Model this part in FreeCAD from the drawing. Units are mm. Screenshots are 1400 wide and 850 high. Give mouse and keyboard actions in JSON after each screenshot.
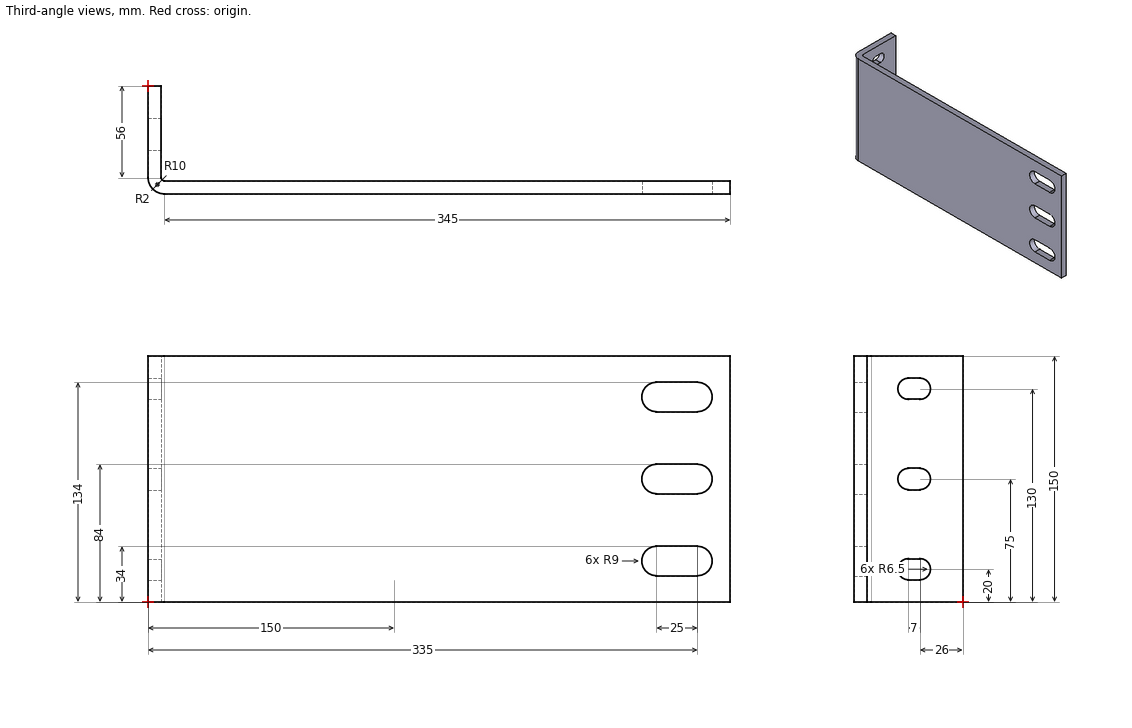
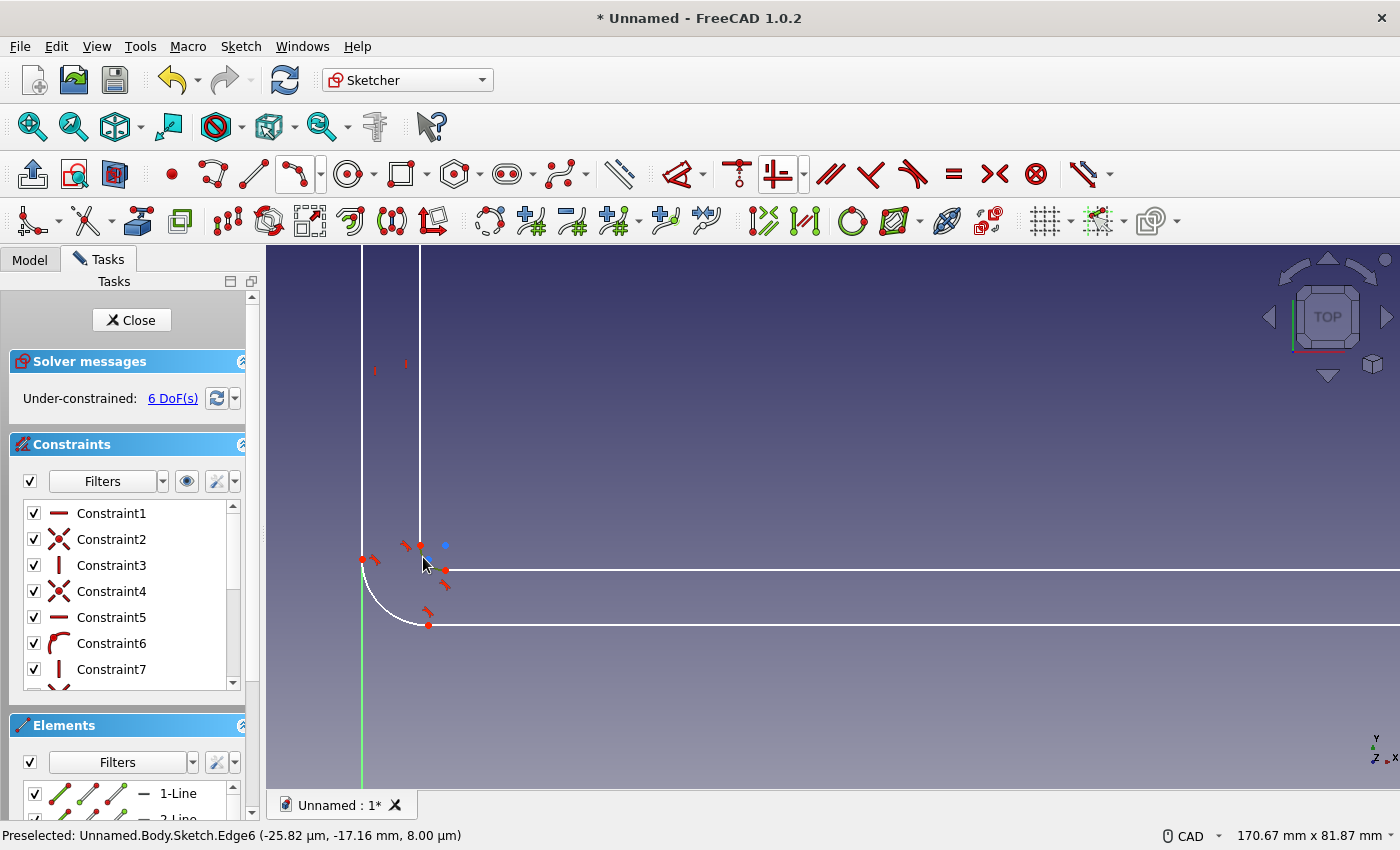
{"action": "left_click", "coordinate": [398, 618]}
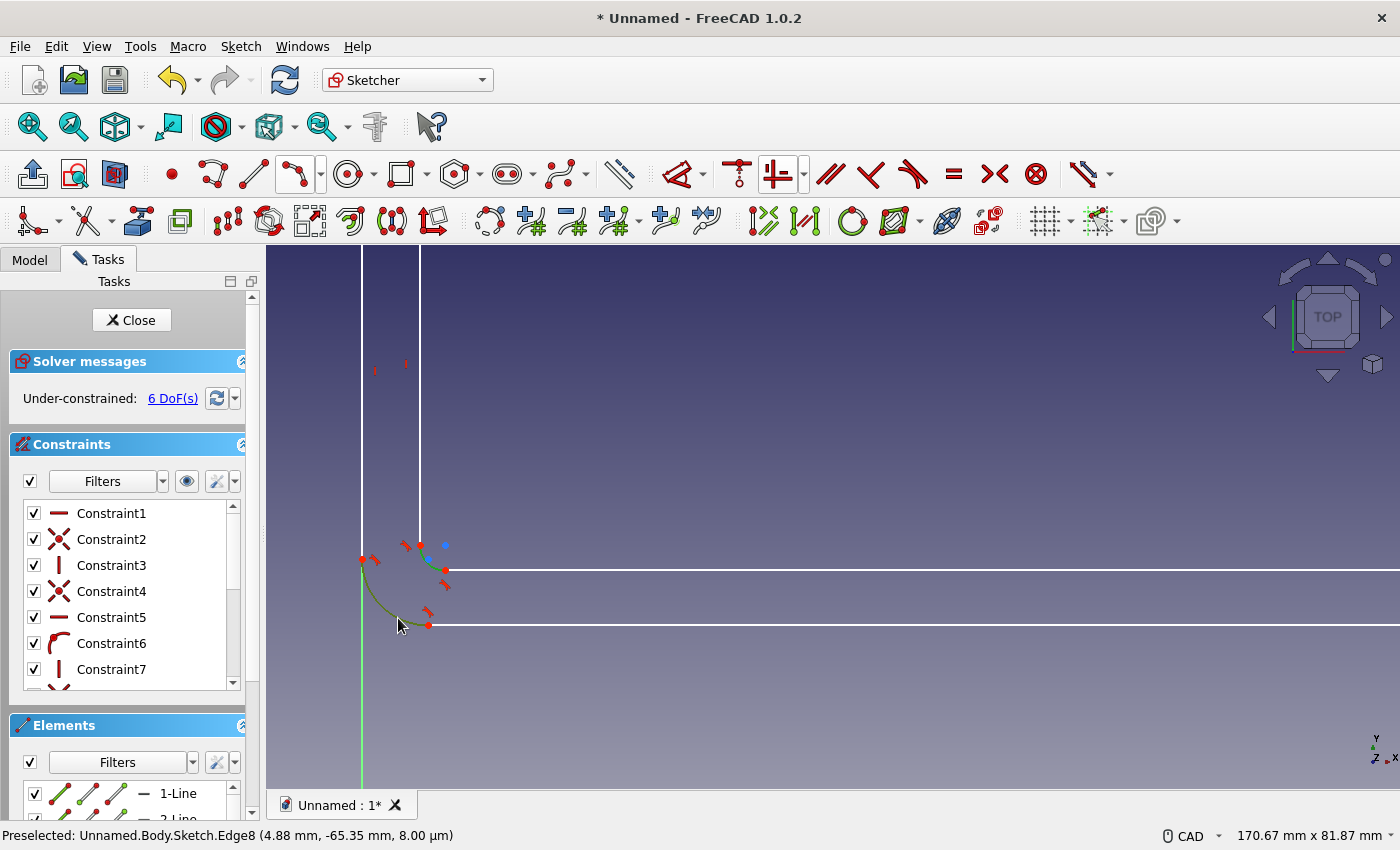
{"action": "left_click", "coordinate": [737, 174]}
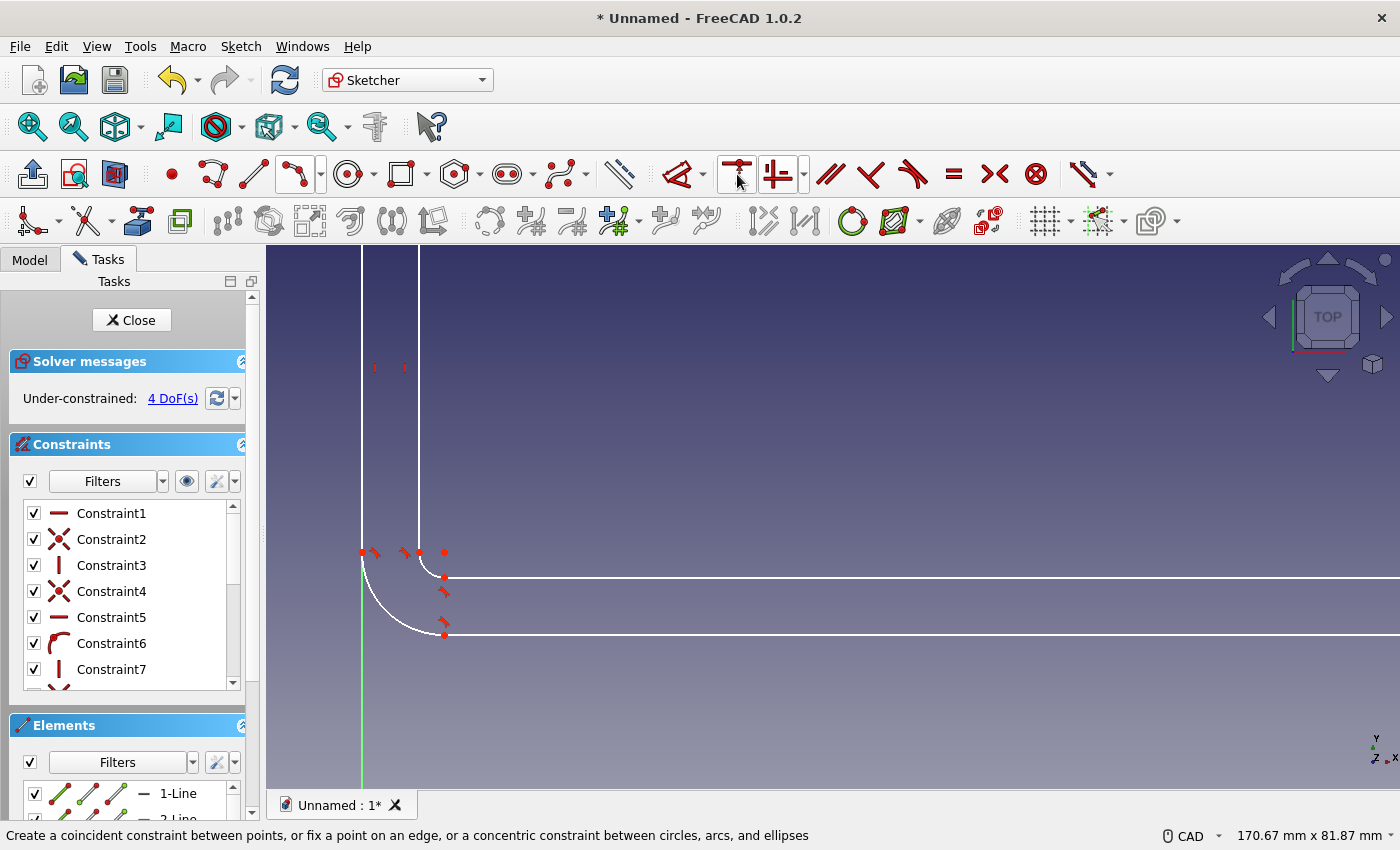
{"action": "left_click", "coordinate": [676, 174]}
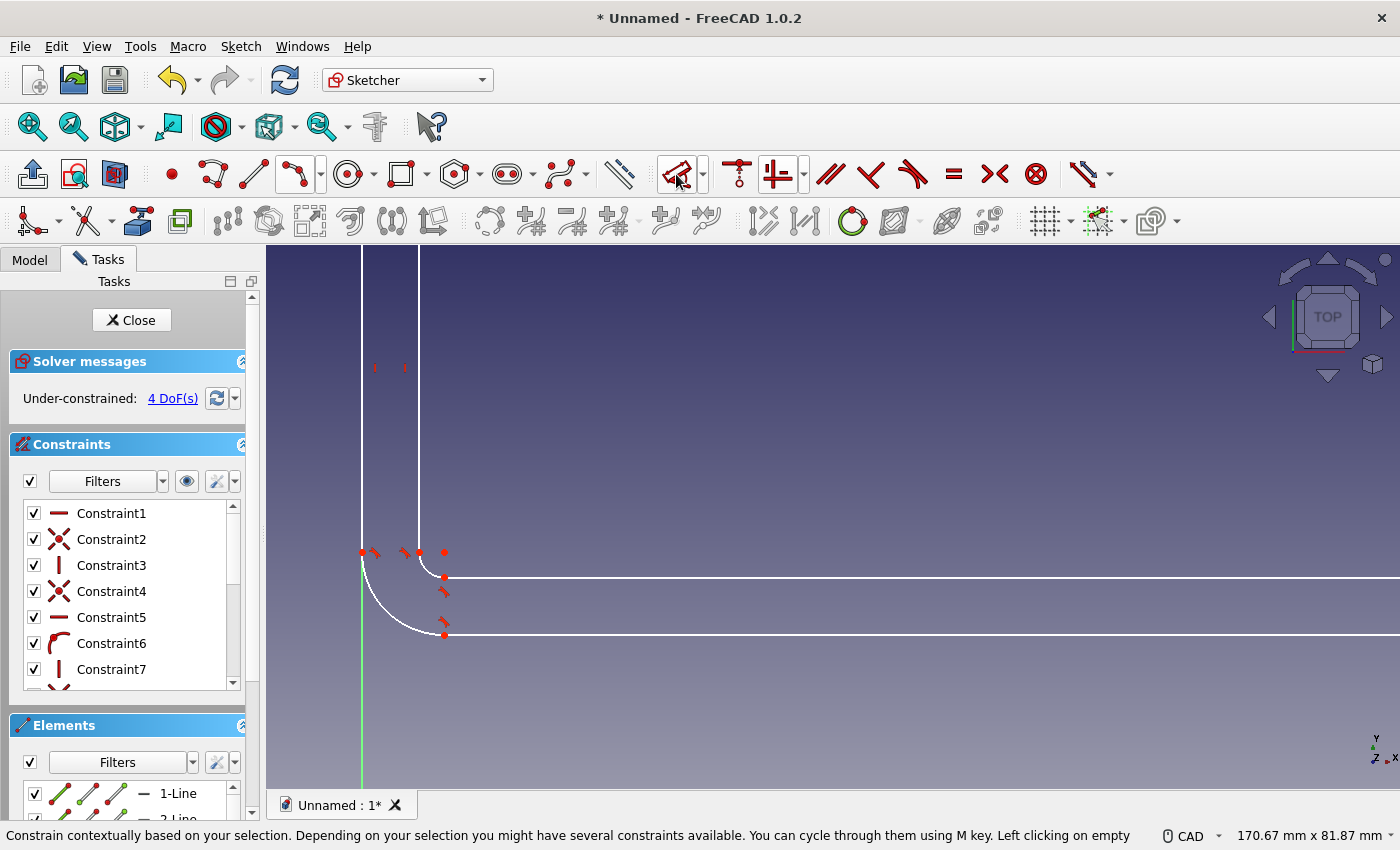
{"action": "scroll", "coordinate": [422, 564], "scroll_direction": "up", "scroll_amount": 6}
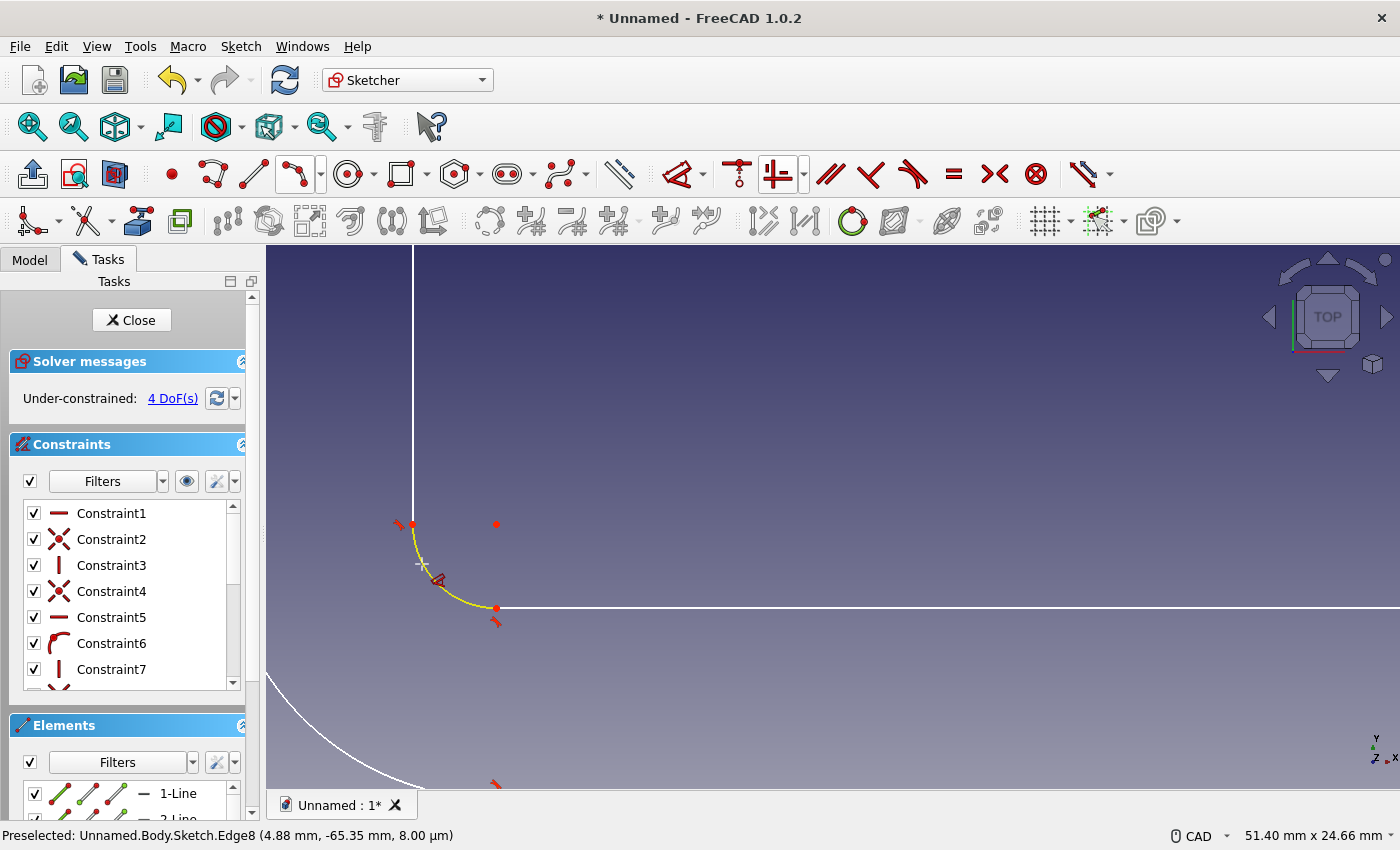
{"action": "left_click", "coordinate": [422, 562]}
{"action": "left_click", "coordinate": [393, 576]}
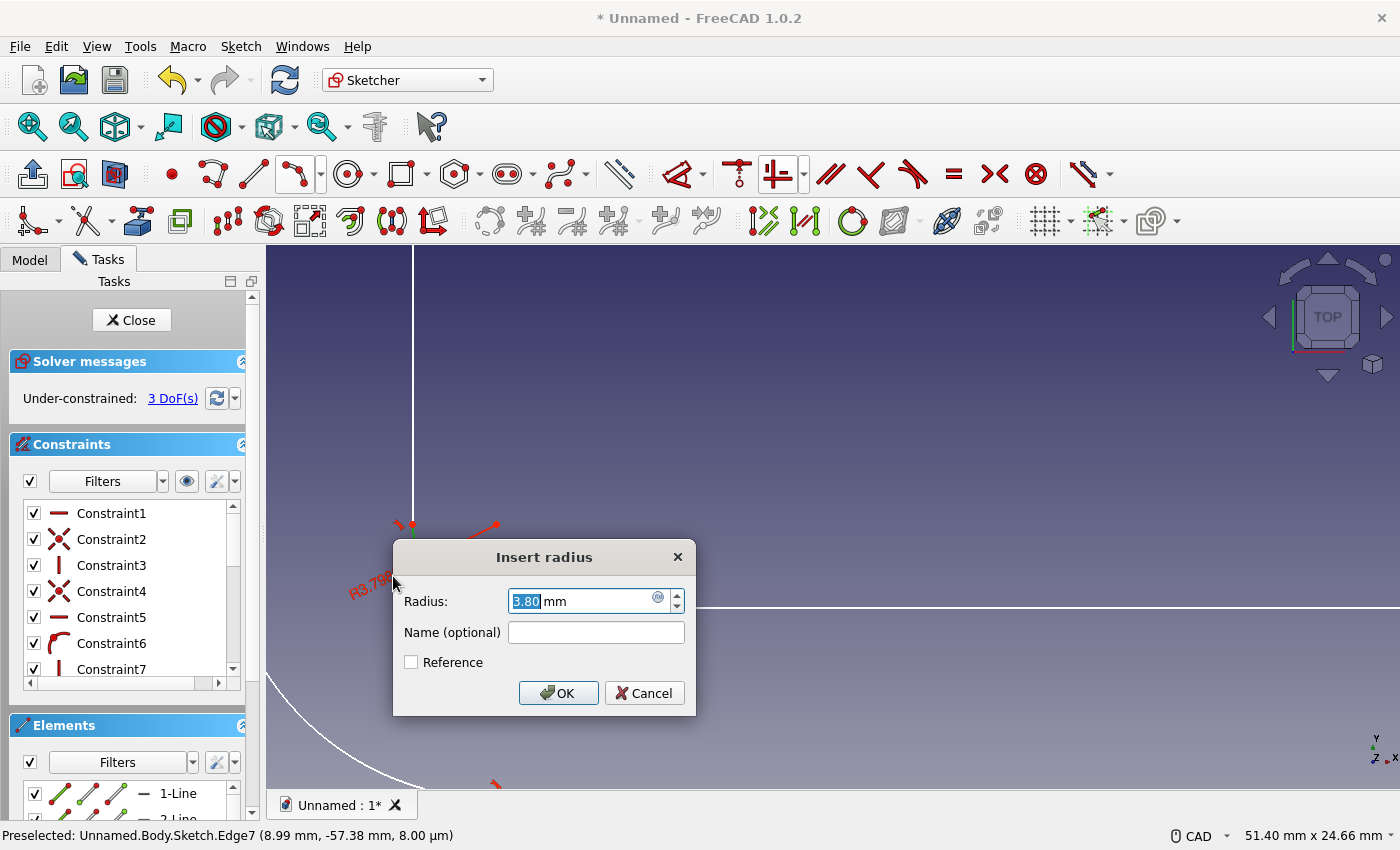
{"action": "type", "text": "2"}
{"action": "key", "text": "Return"}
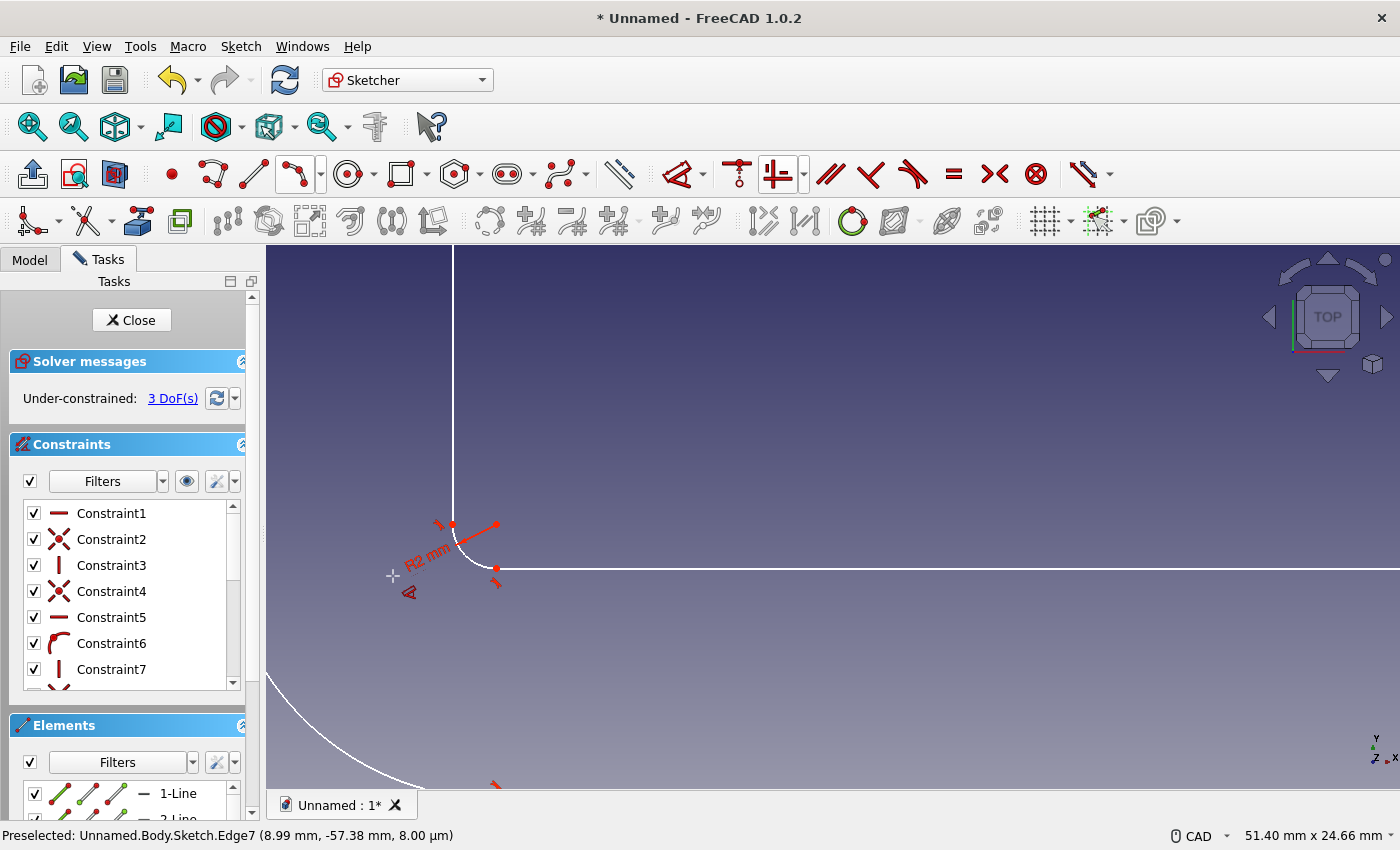
{"action": "scroll", "coordinate": [428, 566], "scroll_direction": "down", "scroll_amount": 12}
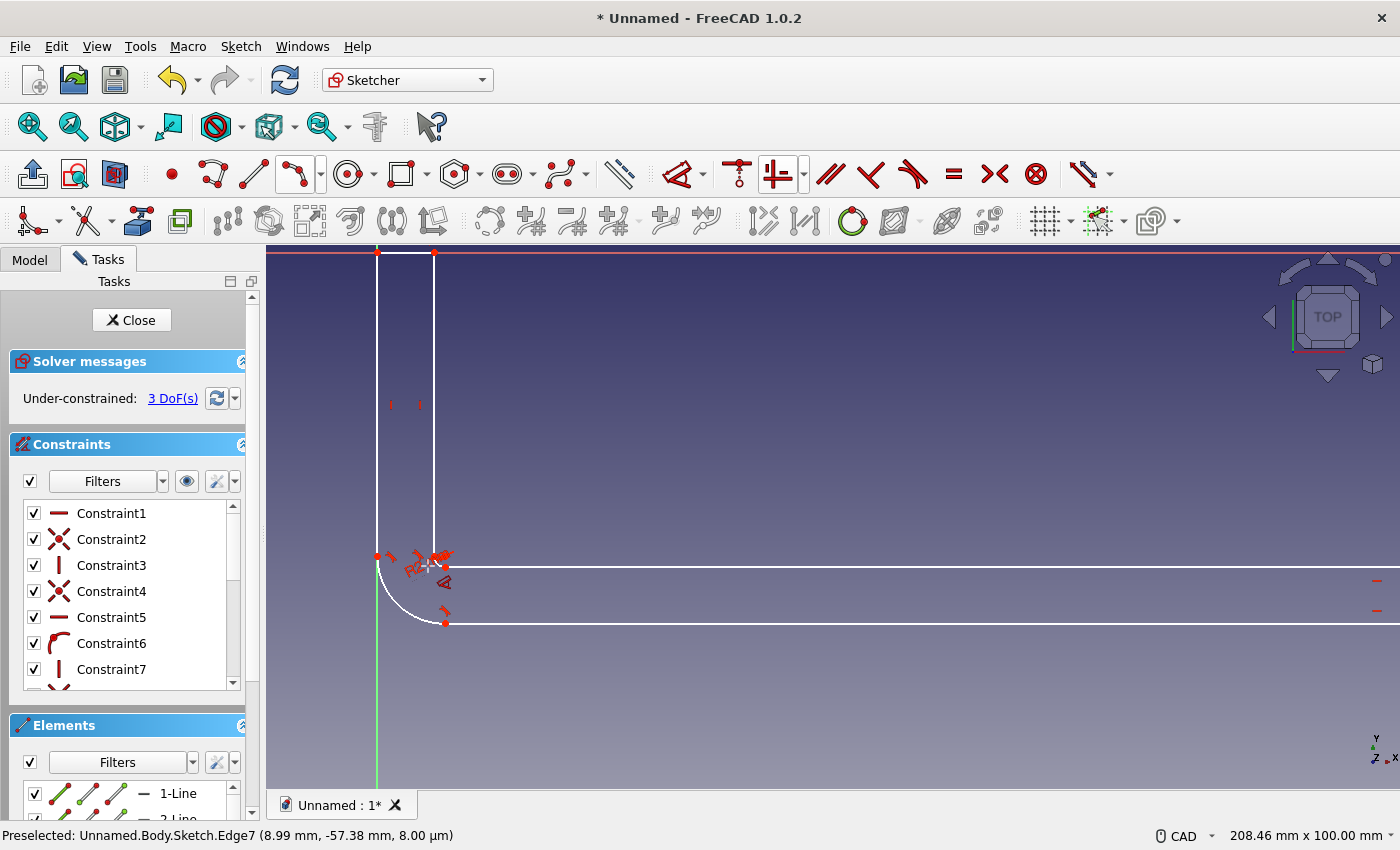
{"action": "scroll", "coordinate": [417, 580], "scroll_direction": "up", "scroll_amount": 4}